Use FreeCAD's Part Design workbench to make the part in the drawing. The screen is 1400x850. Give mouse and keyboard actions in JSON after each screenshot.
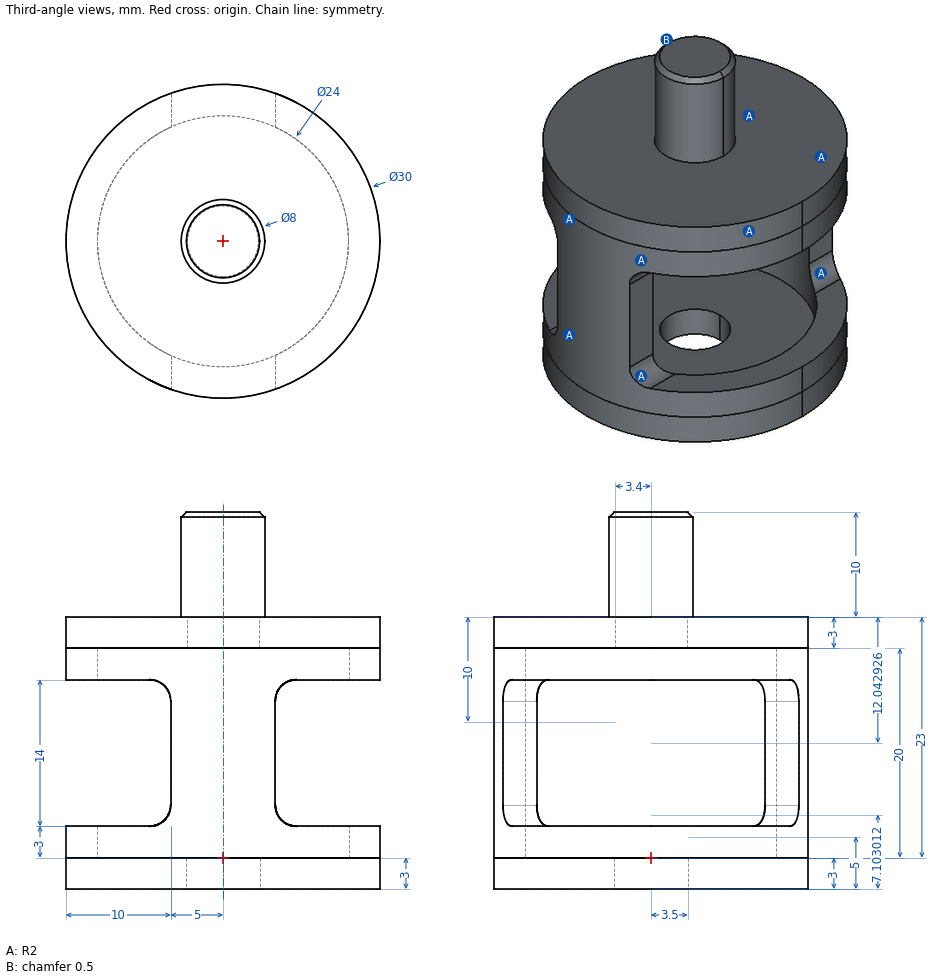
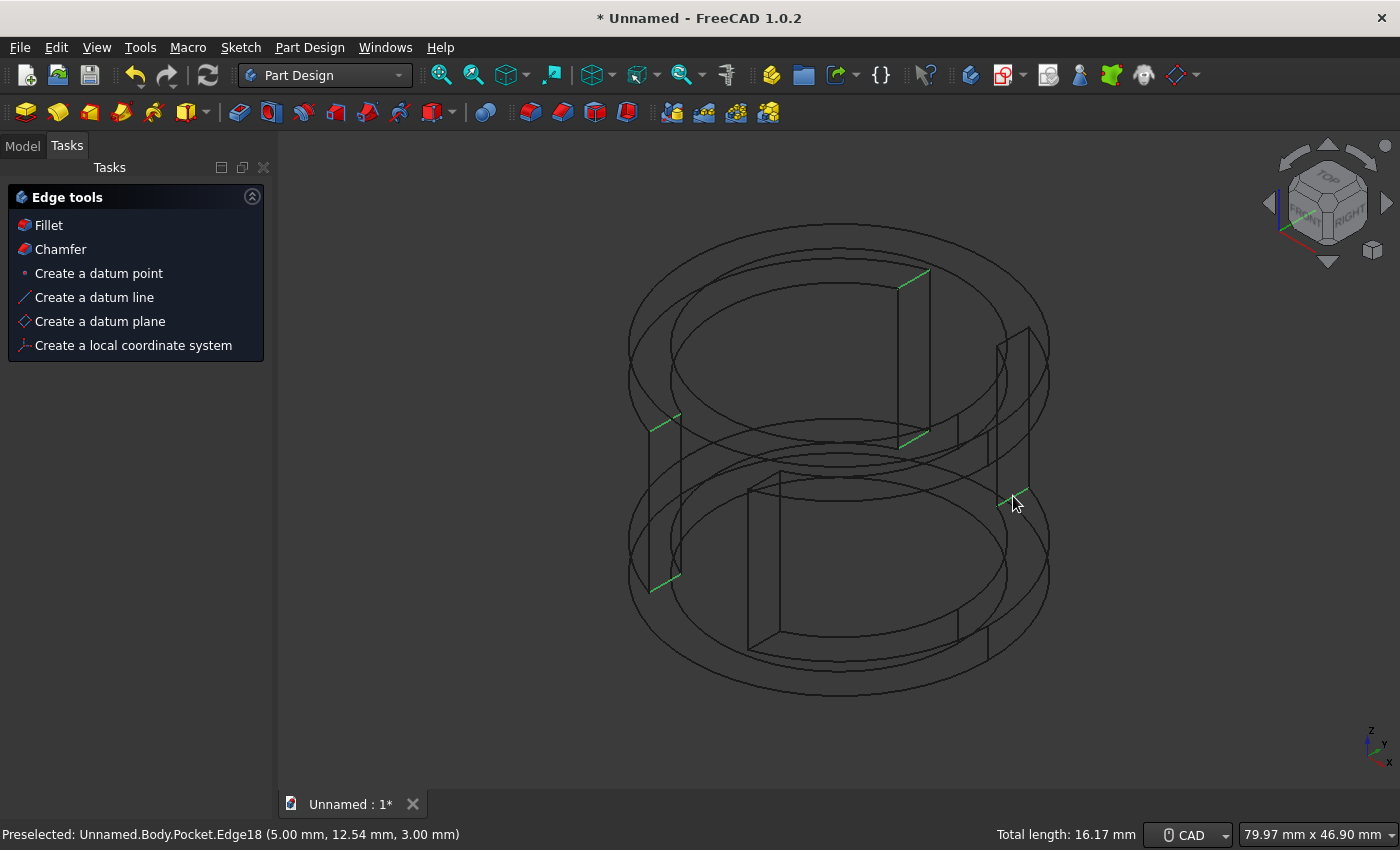
{"action": "left_click", "coordinate": [764, 640], "text": "ctrl"}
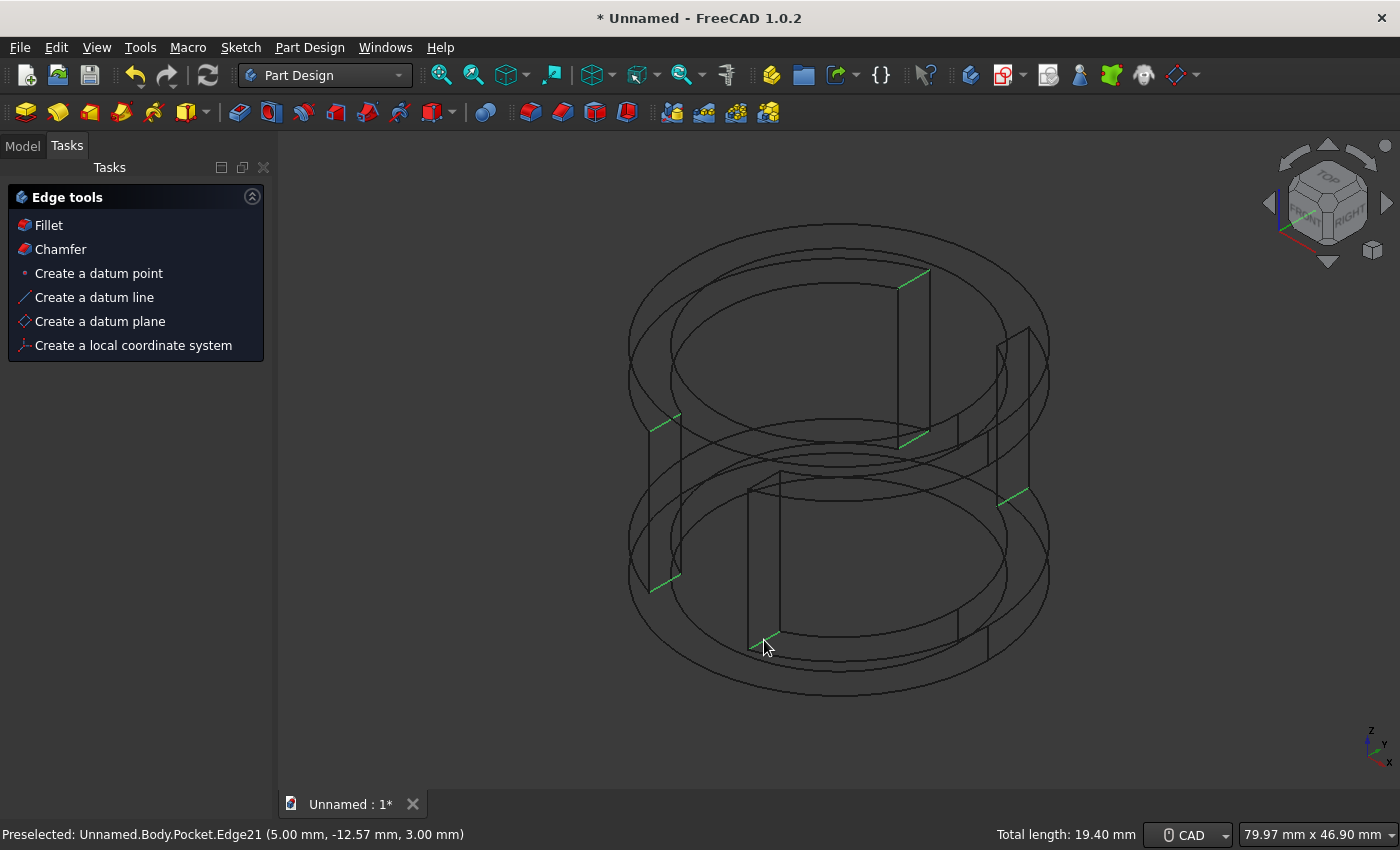
{"action": "left_click", "coordinate": [1013, 336], "text": "ctrl"}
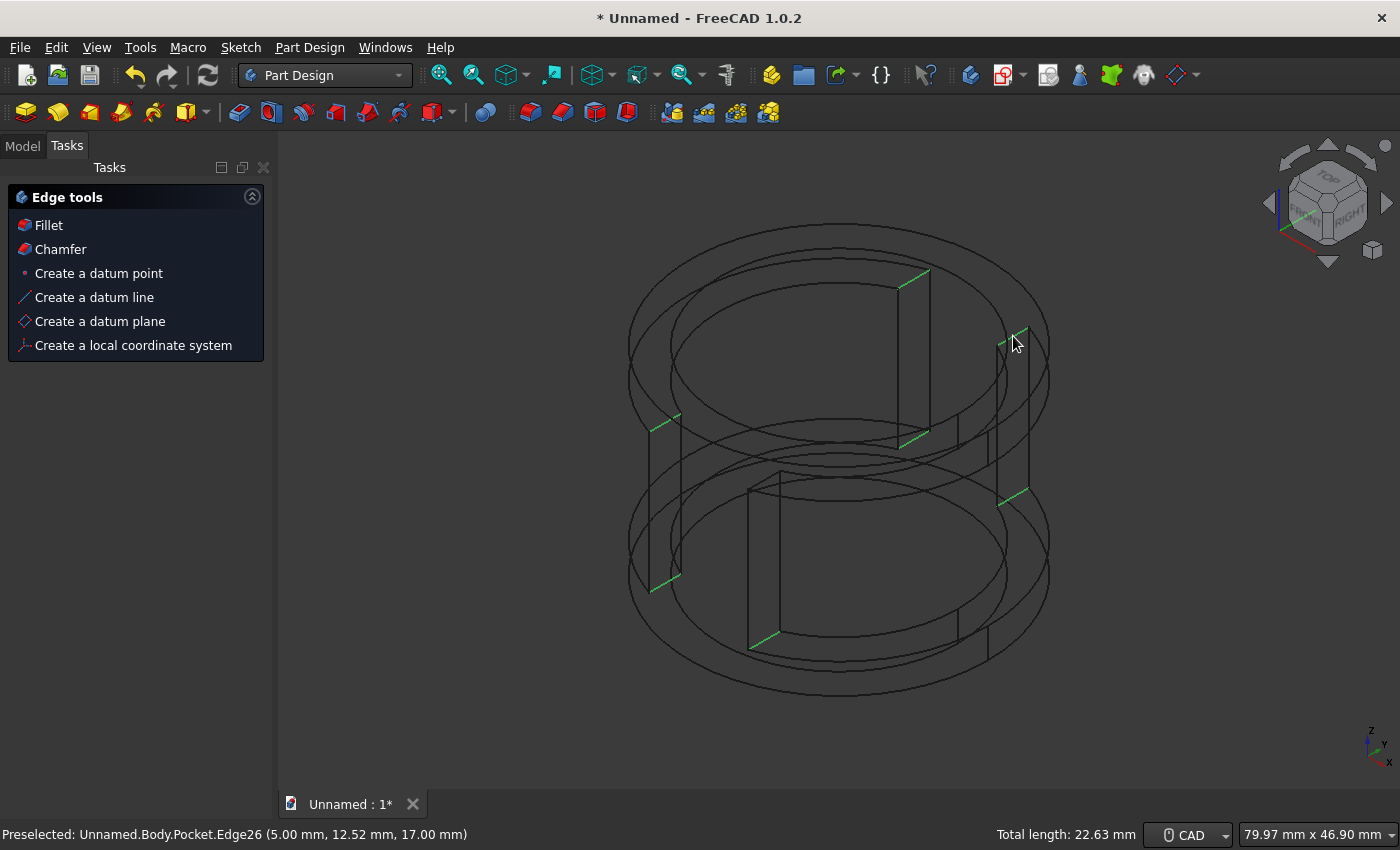
{"action": "left_click", "coordinate": [764, 479], "text": "ctrl"}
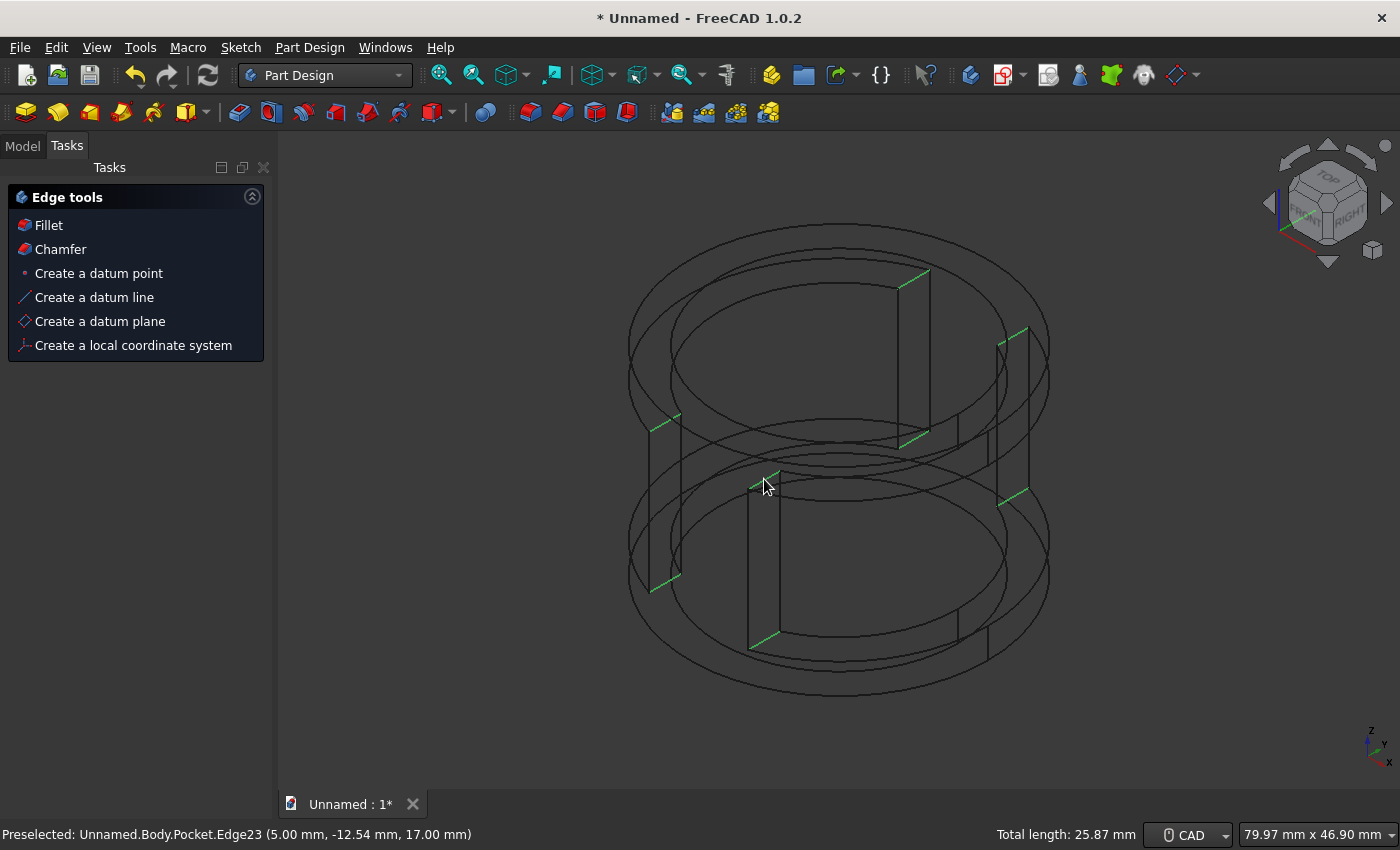
{"action": "key", "text": "v 1"}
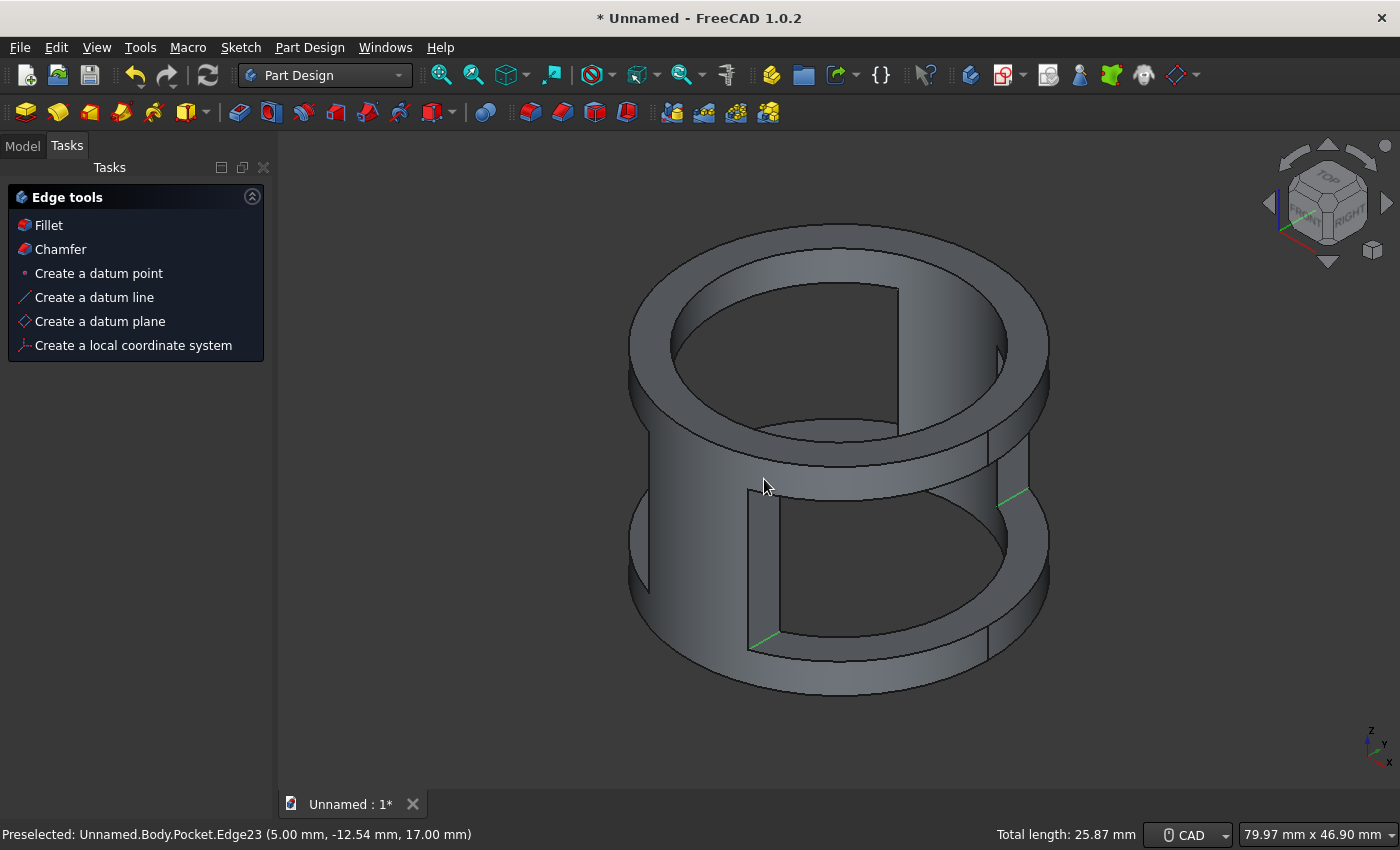
{"action": "left_click", "coordinate": [532, 112]}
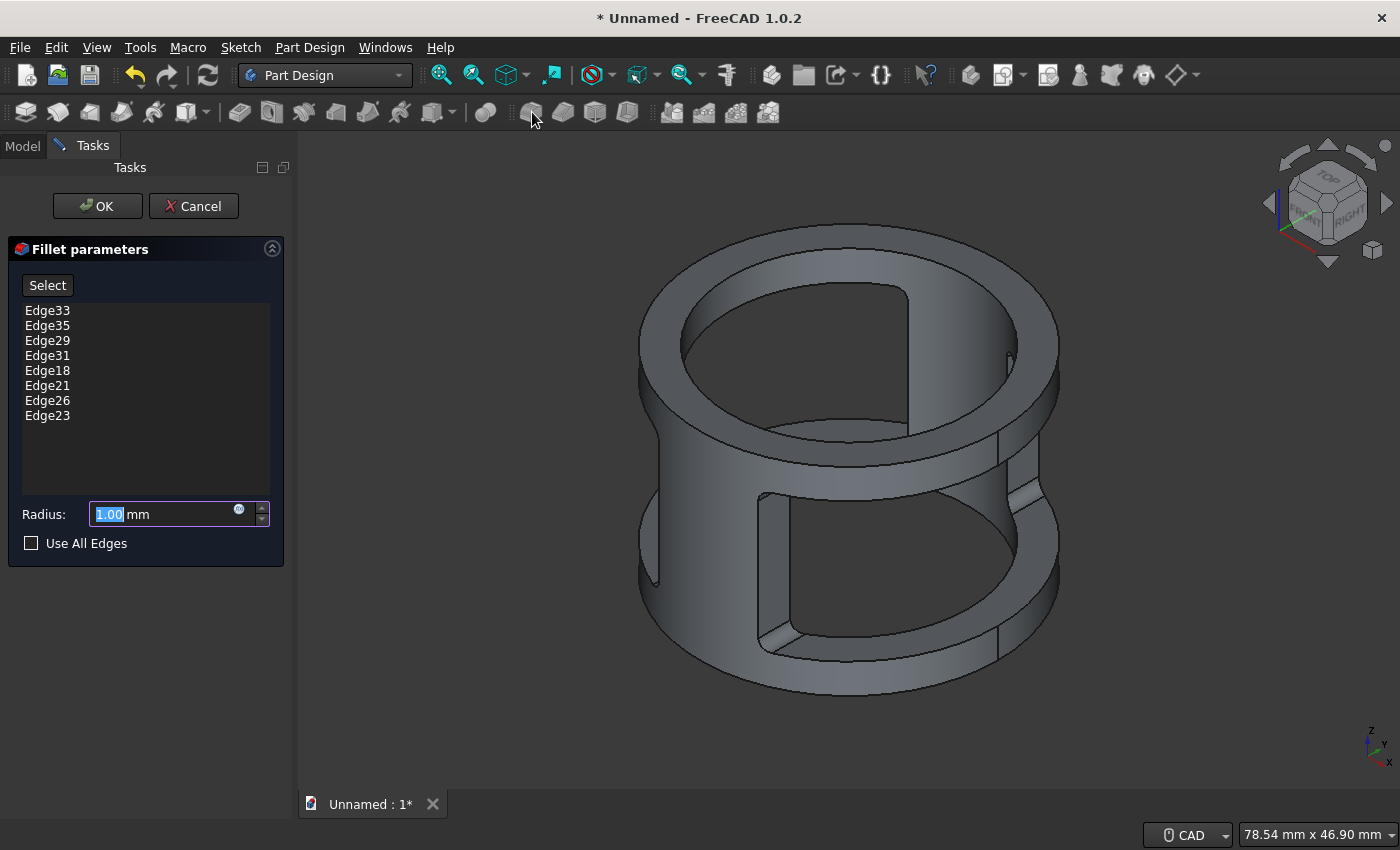
{"action": "type", "text": "2"}
{"action": "key", "text": "Tab"}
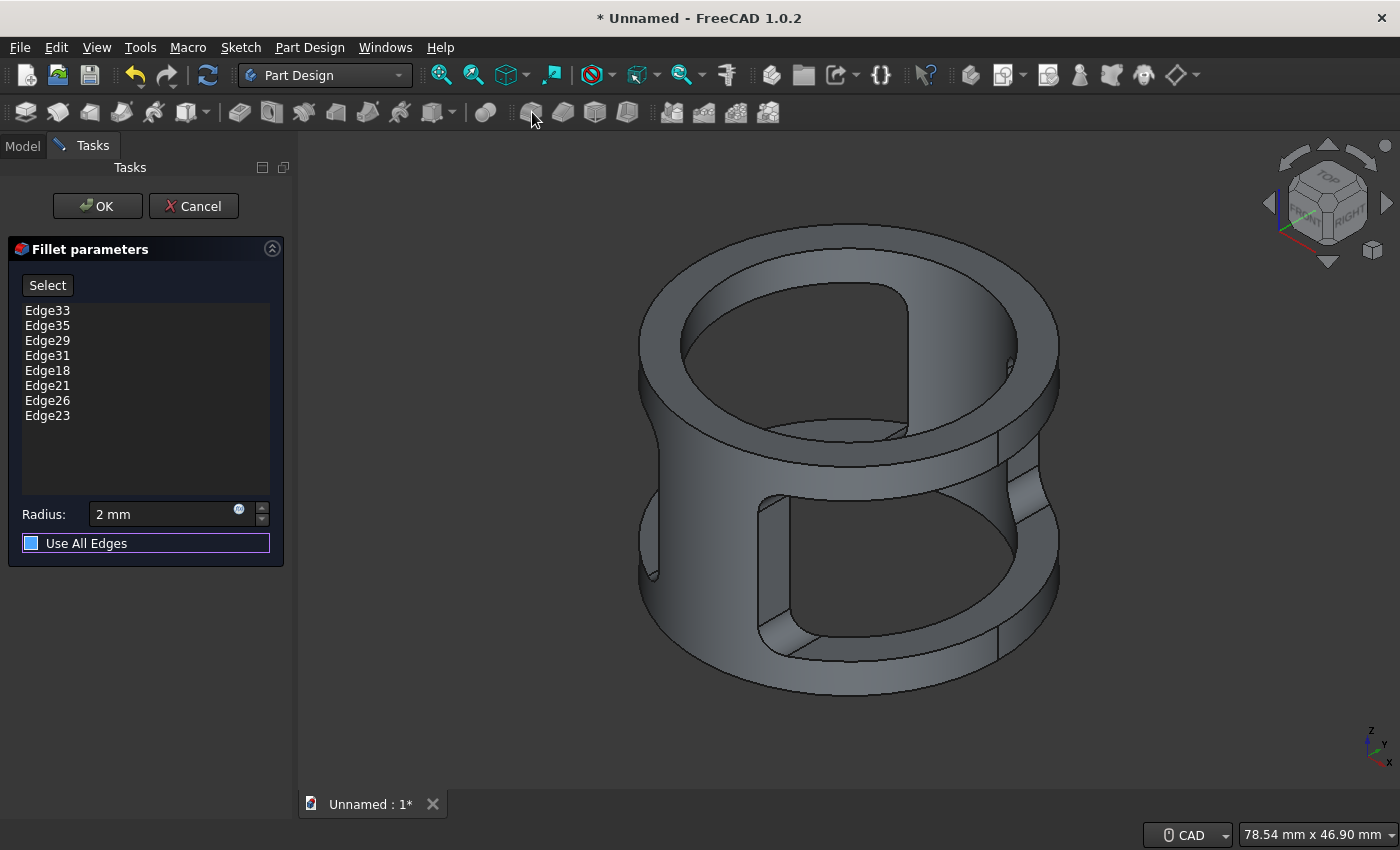
{"action": "left_click", "coordinate": [98, 206]}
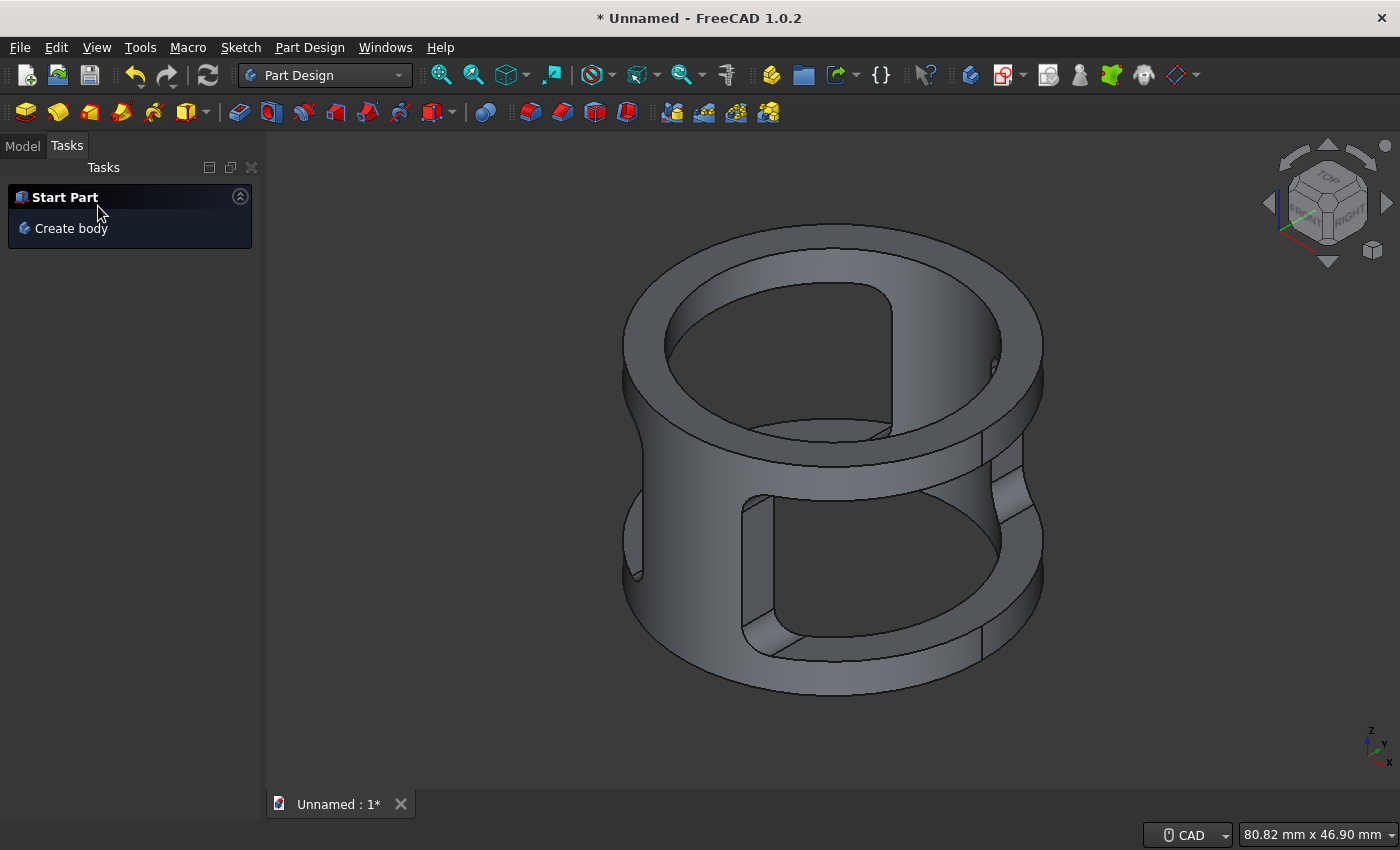
{"action": "left_click", "coordinate": [972, 76]}